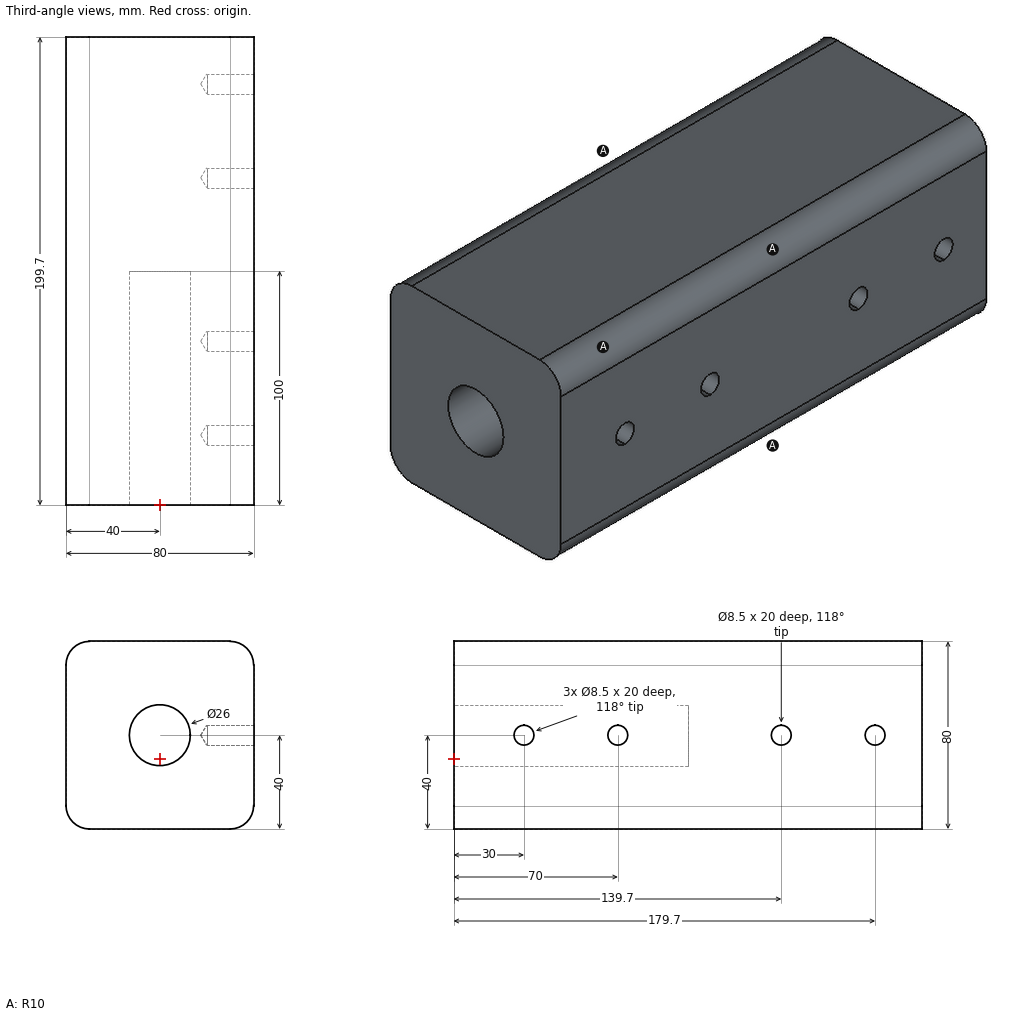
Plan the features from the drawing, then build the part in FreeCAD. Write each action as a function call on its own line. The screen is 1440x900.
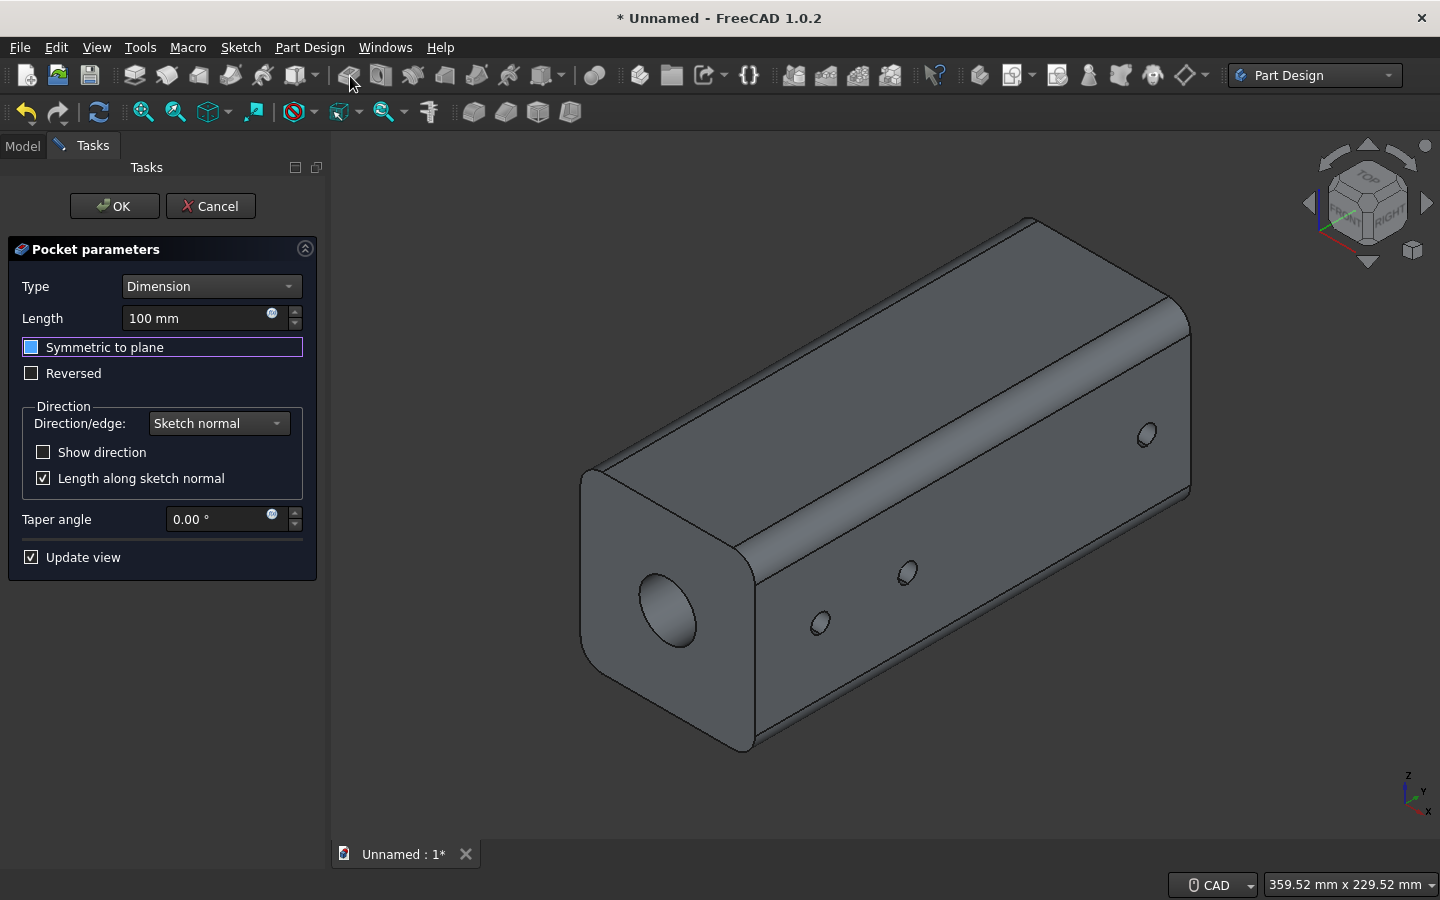
click(115, 206)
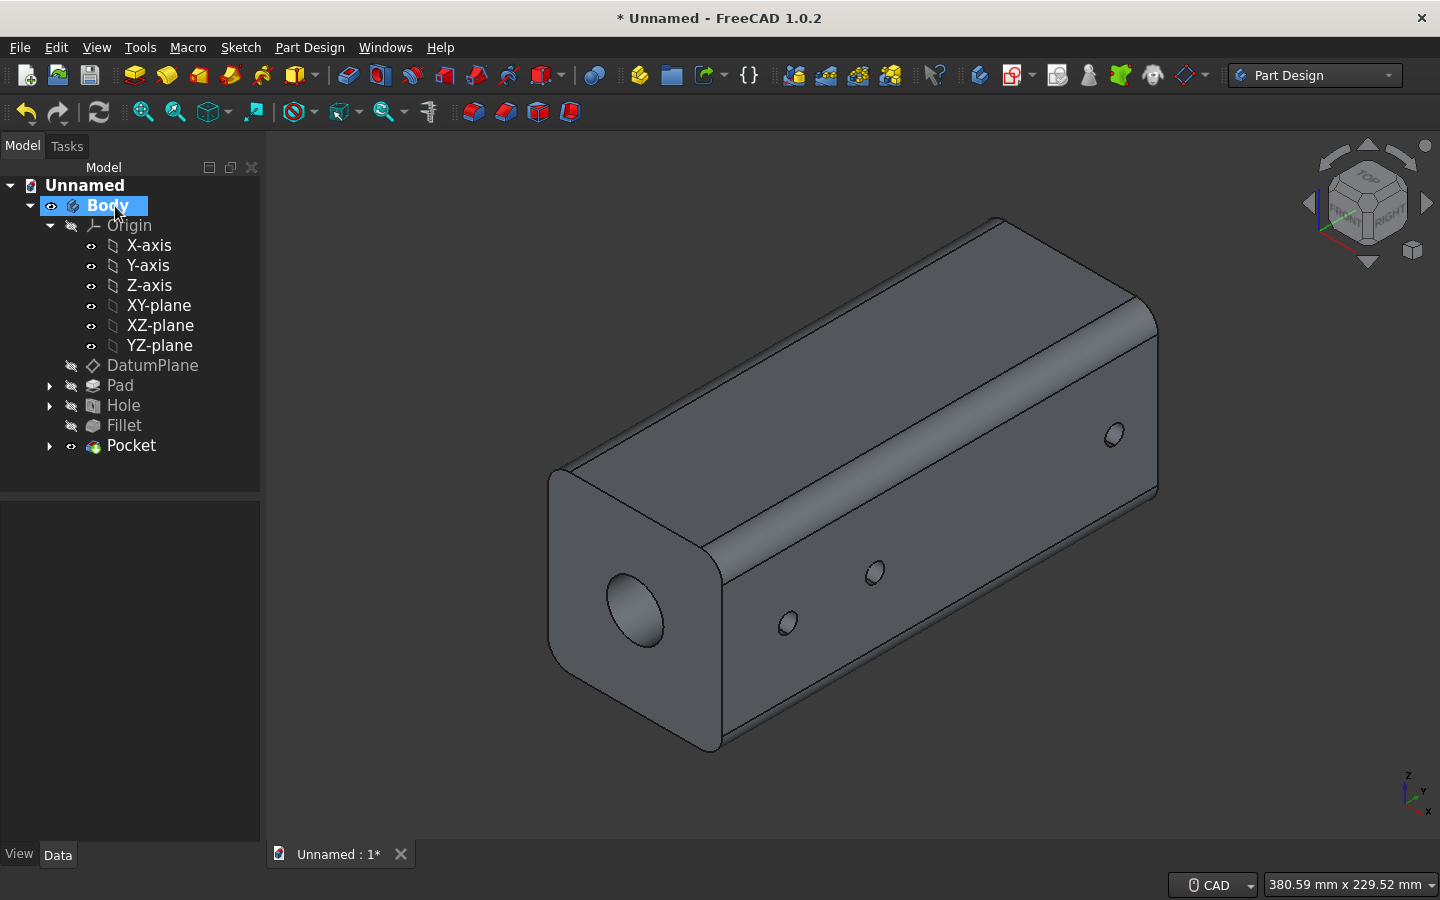
click(1002, 498)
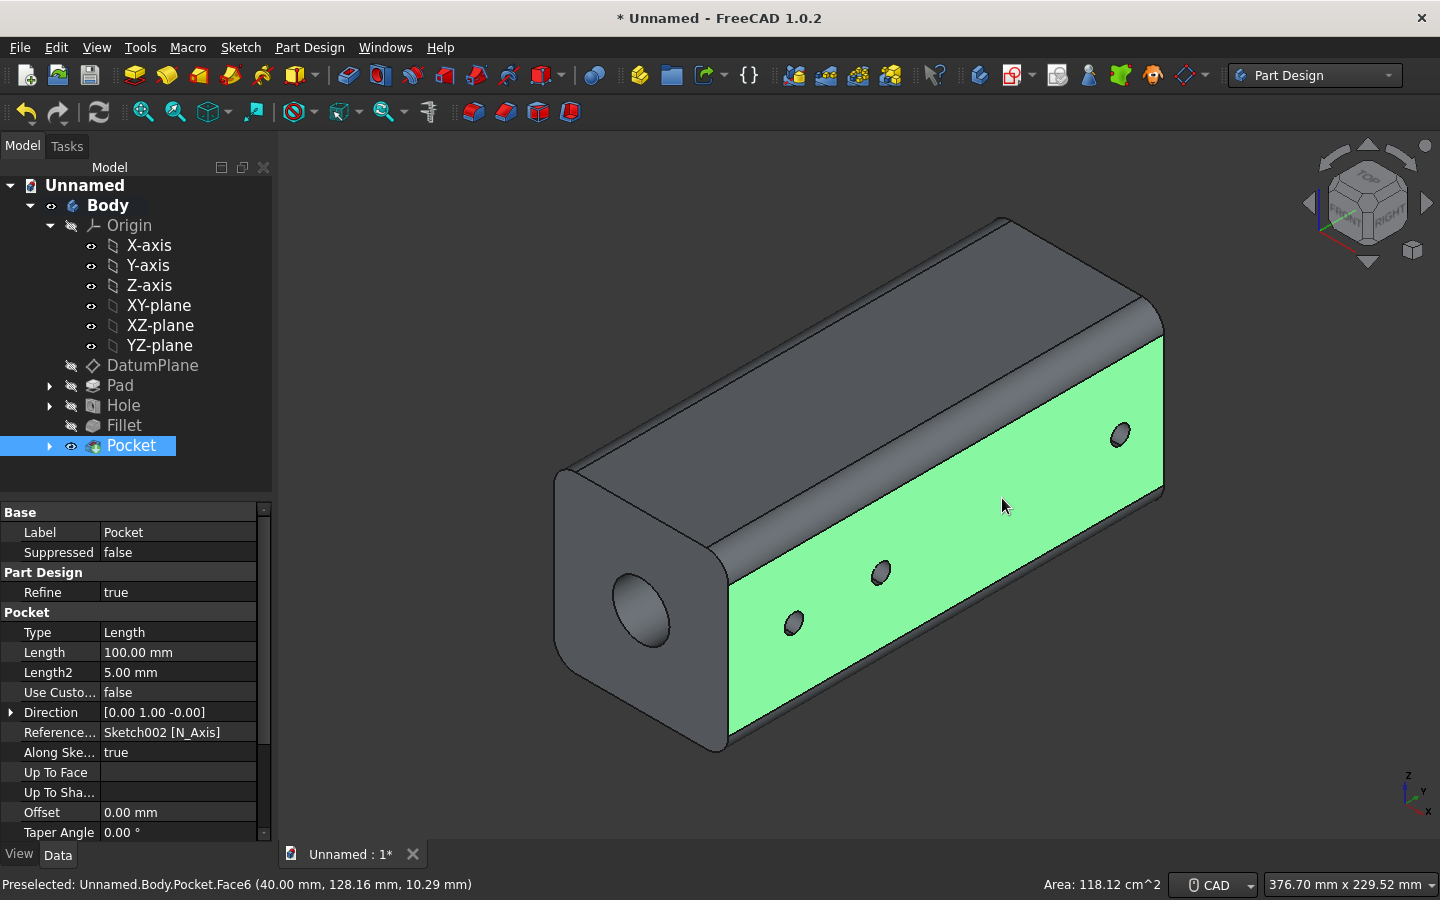
click(1012, 76)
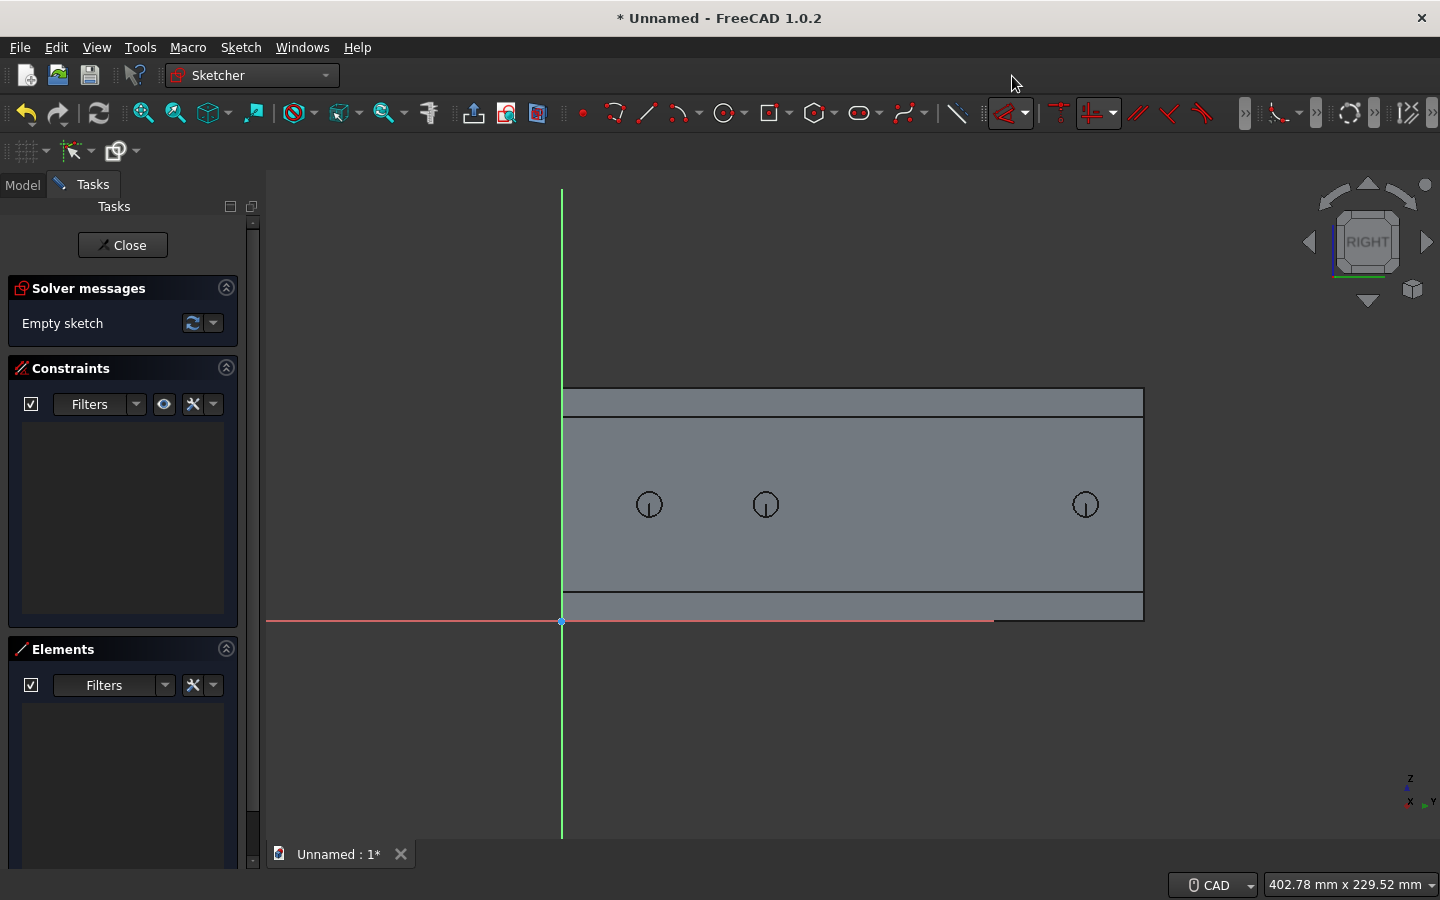
scroll(981, 504, up, 14)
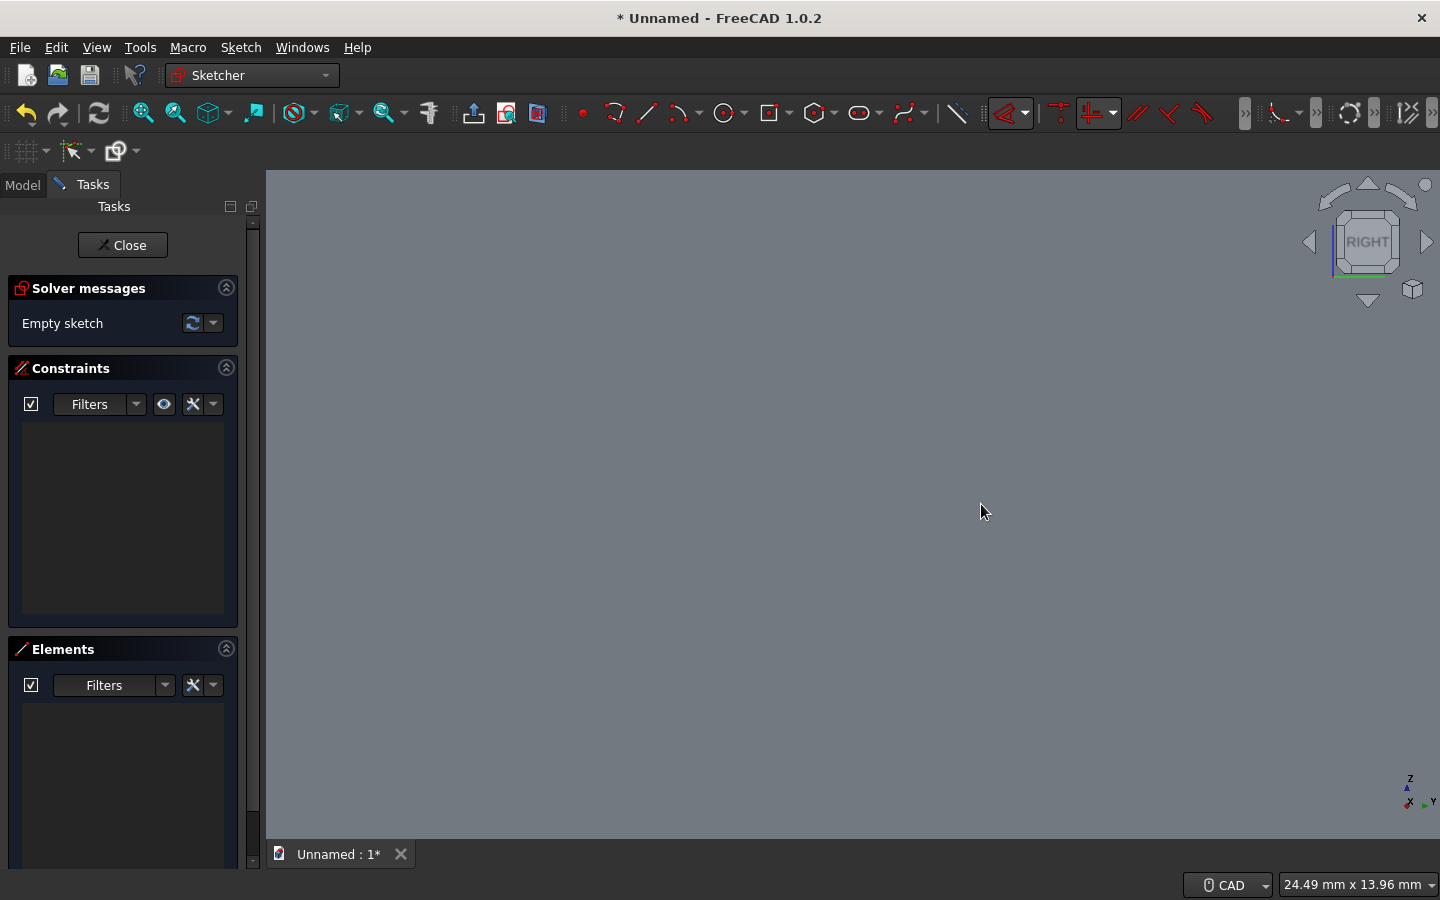
key(g)
key(c)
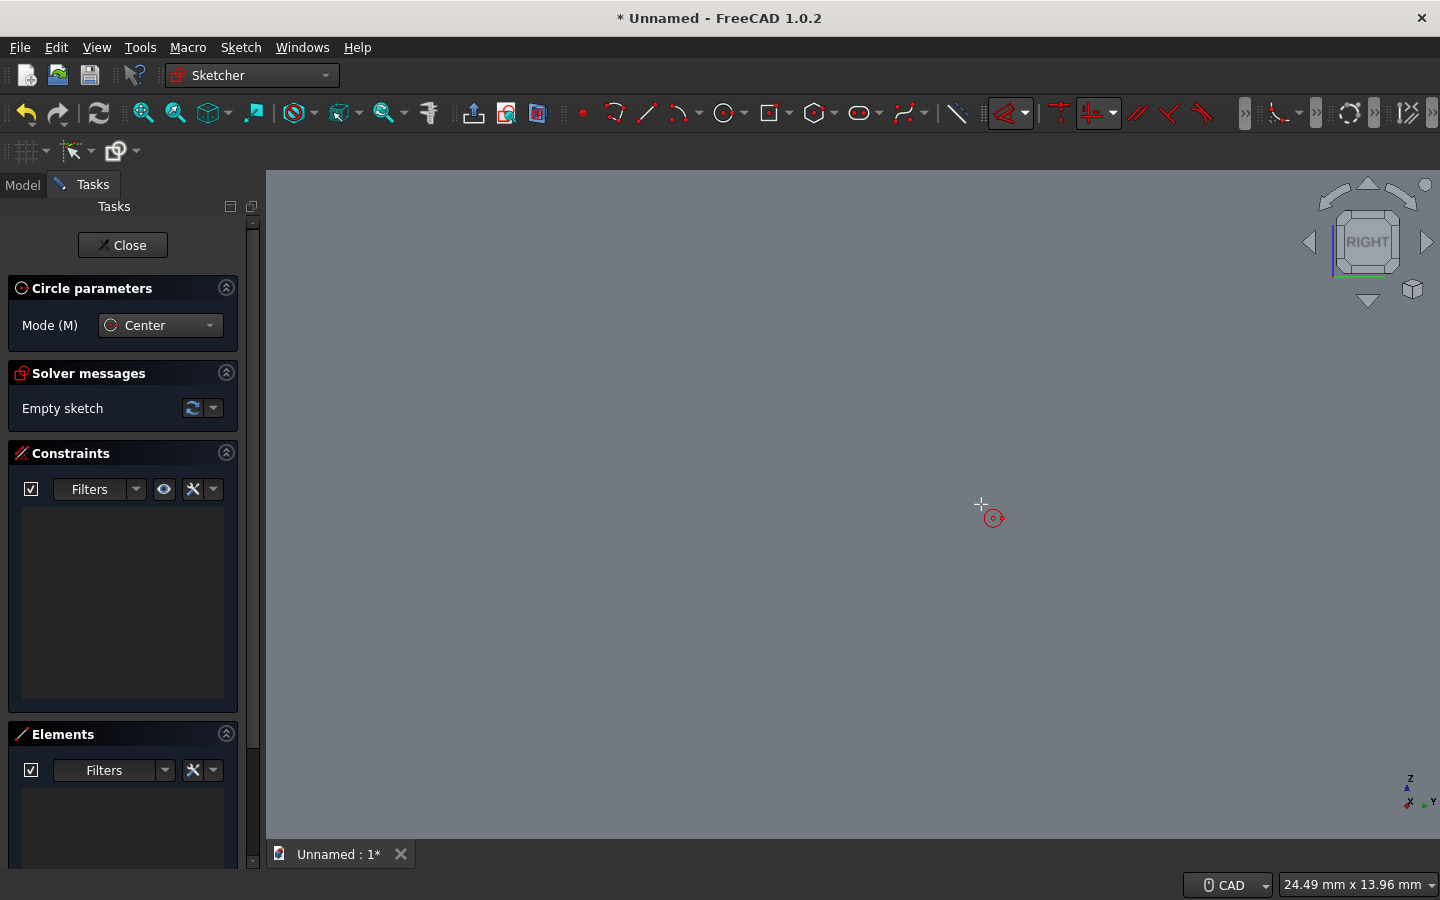
click(777, 504)
click(921, 360)
key(Escape)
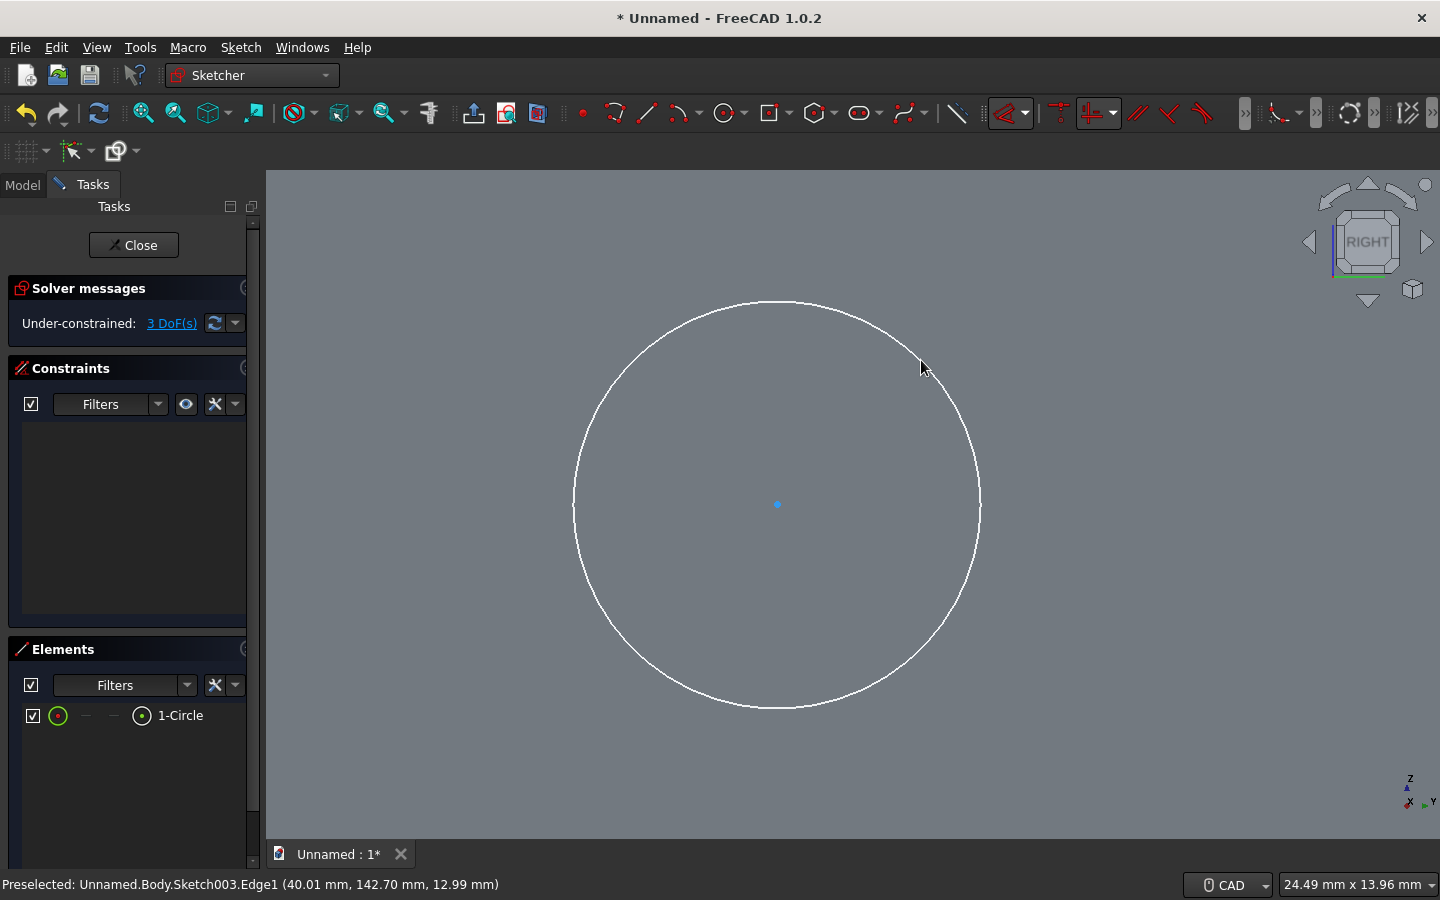
click(921, 361)